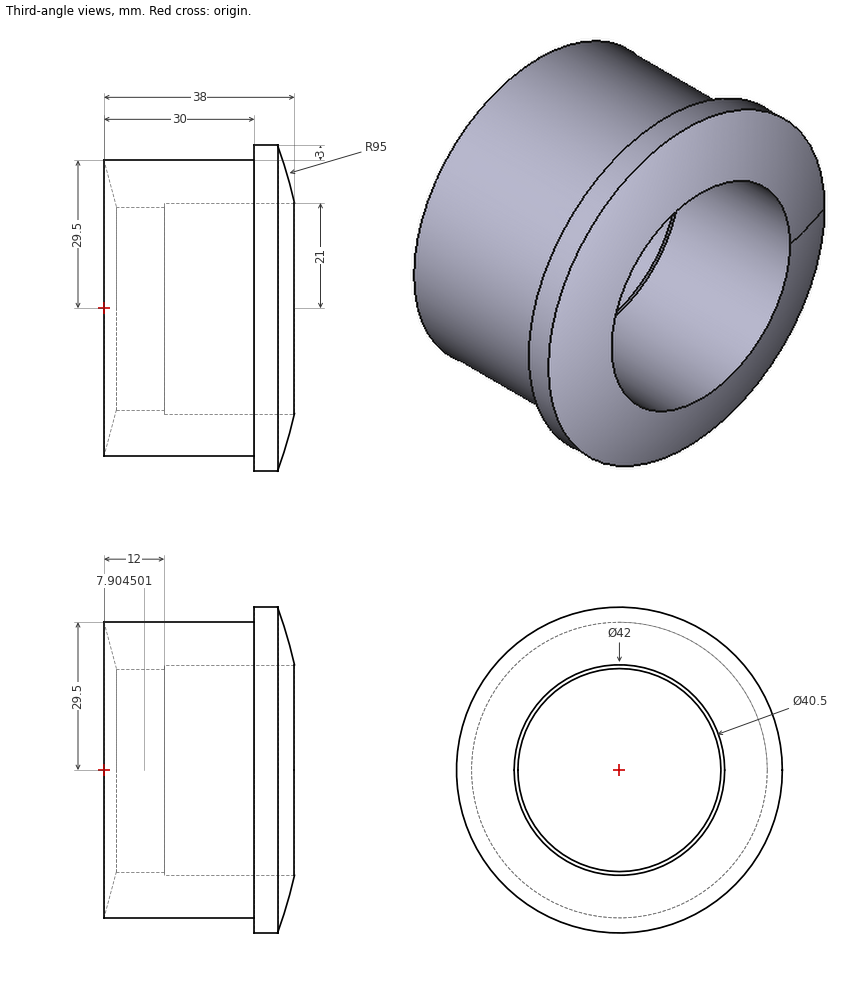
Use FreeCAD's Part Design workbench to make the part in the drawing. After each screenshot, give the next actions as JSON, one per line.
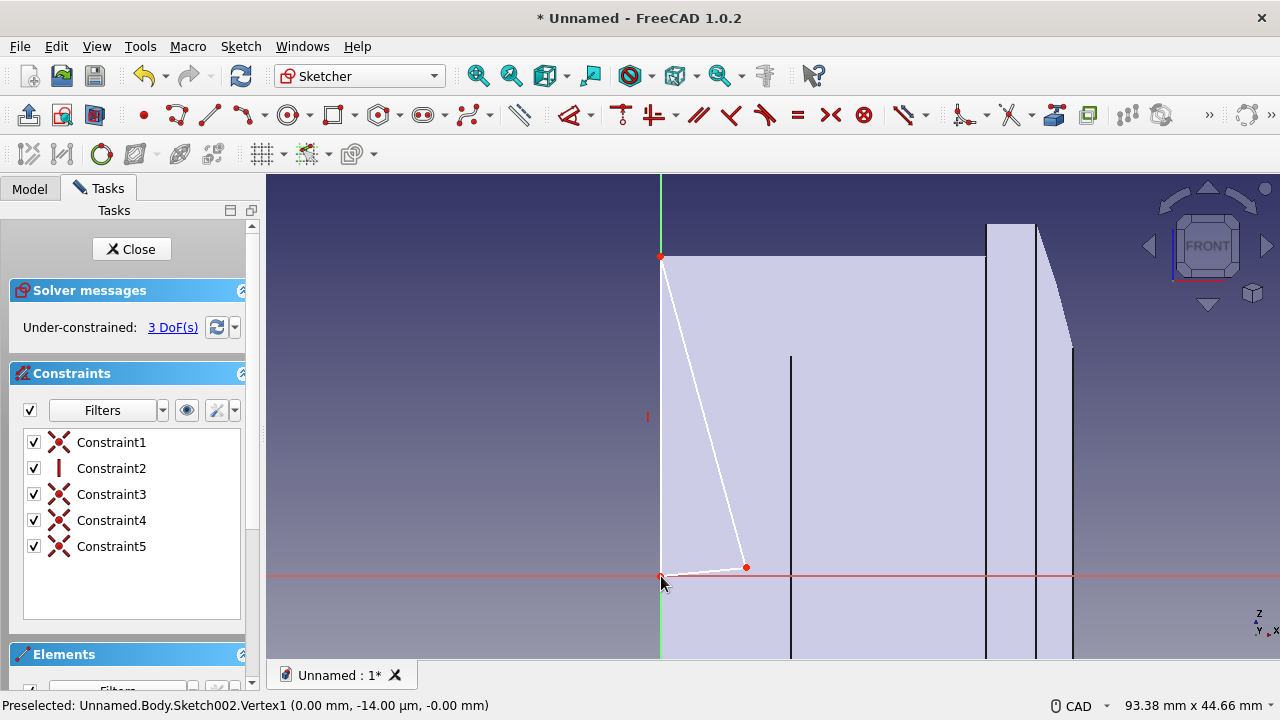
{"action": "left_click", "coordinate": [686, 574]}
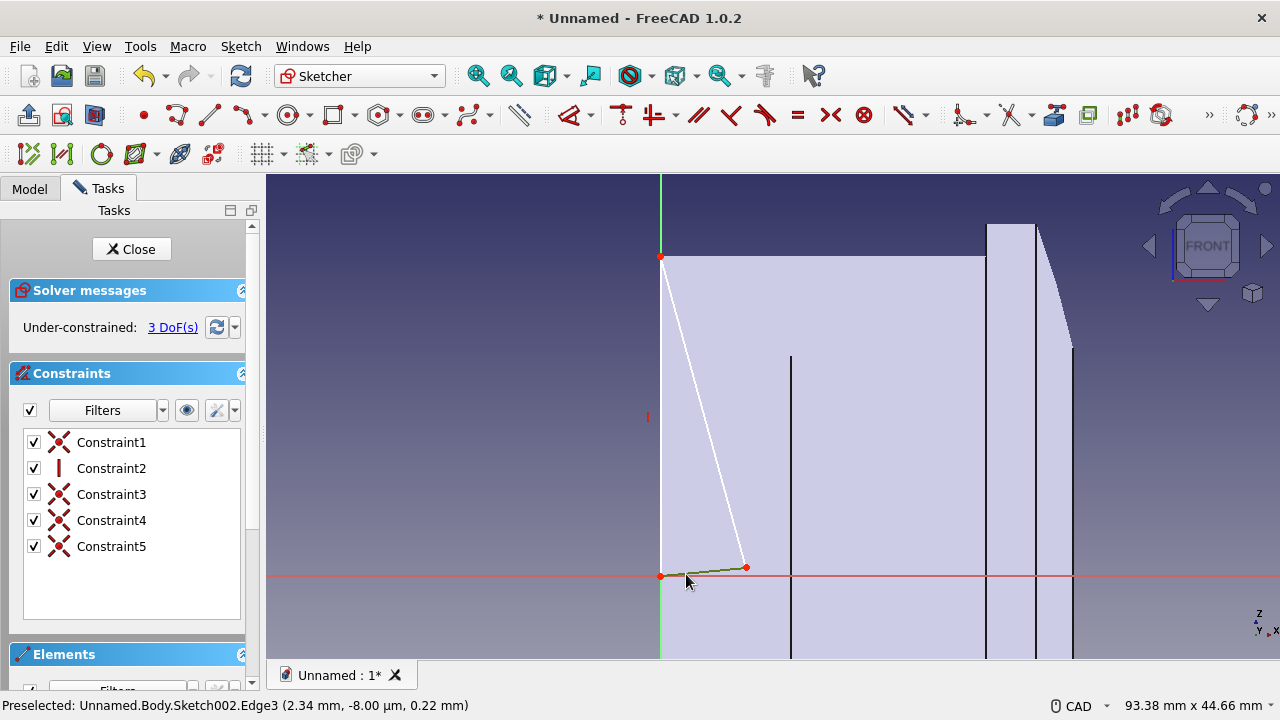
{"action": "left_click", "coordinate": [676, 116]}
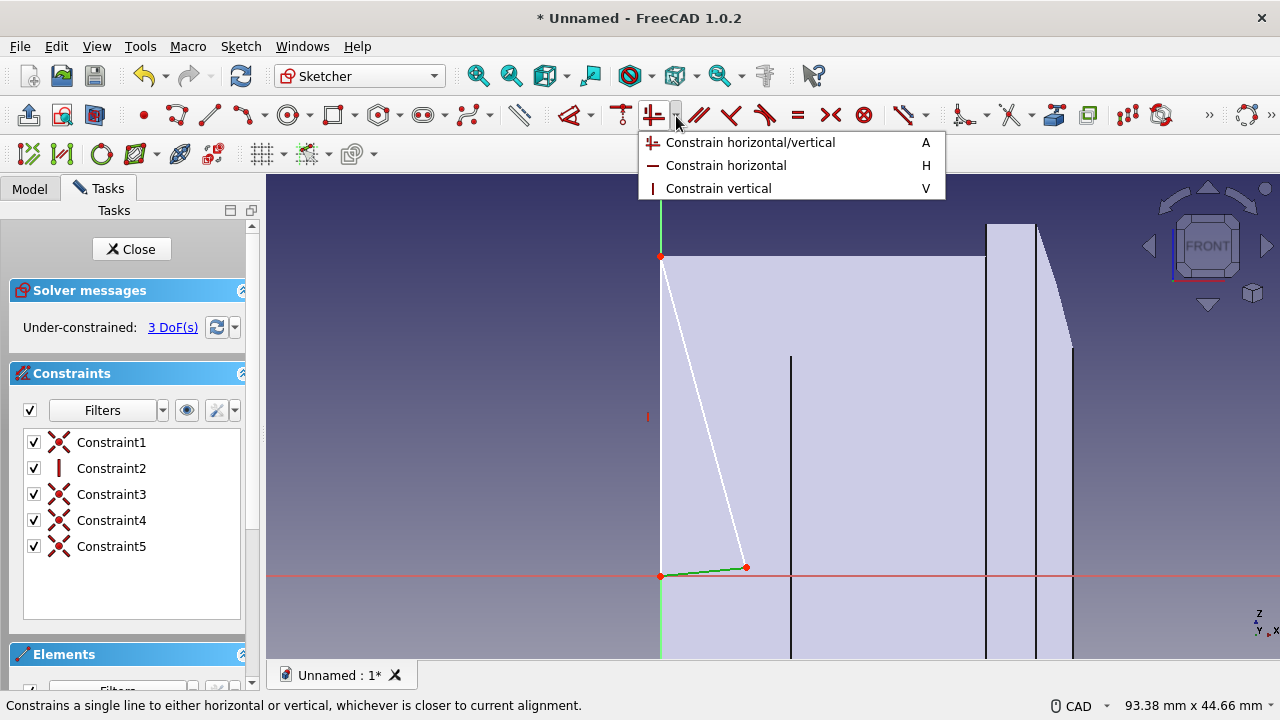
{"action": "left_click", "coordinate": [792, 166]}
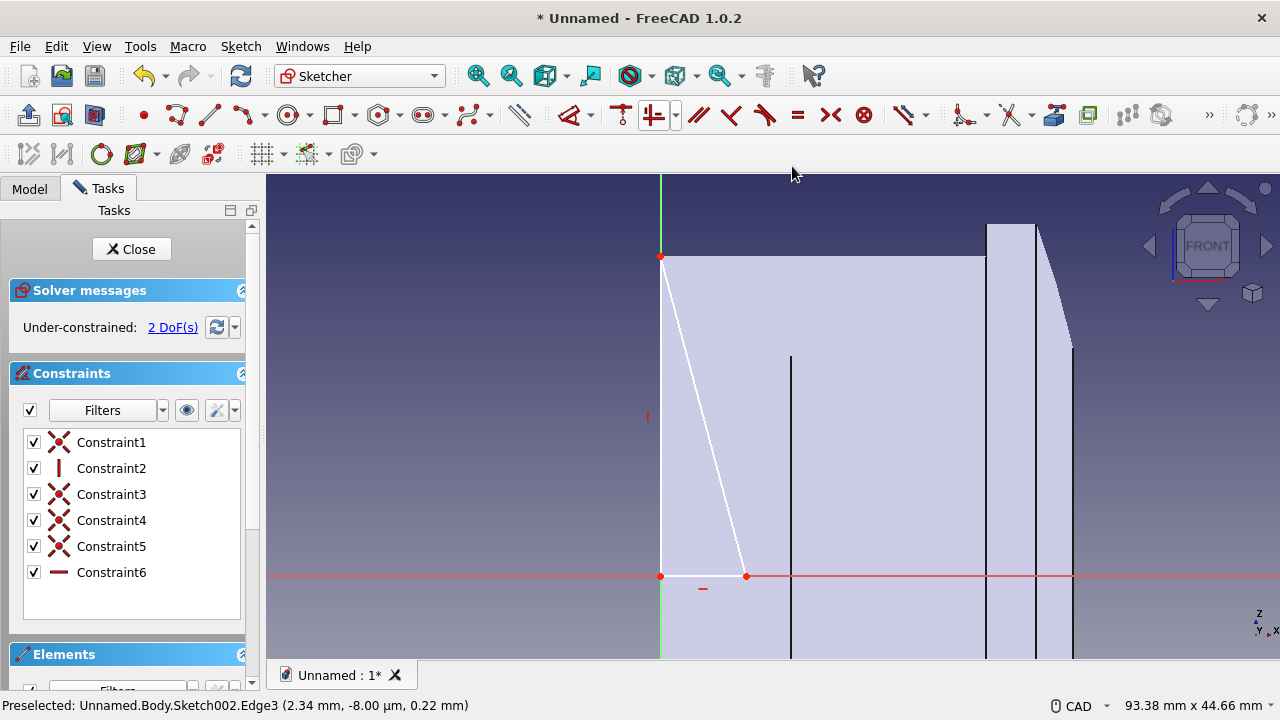
{"action": "left_click", "coordinate": [568, 116]}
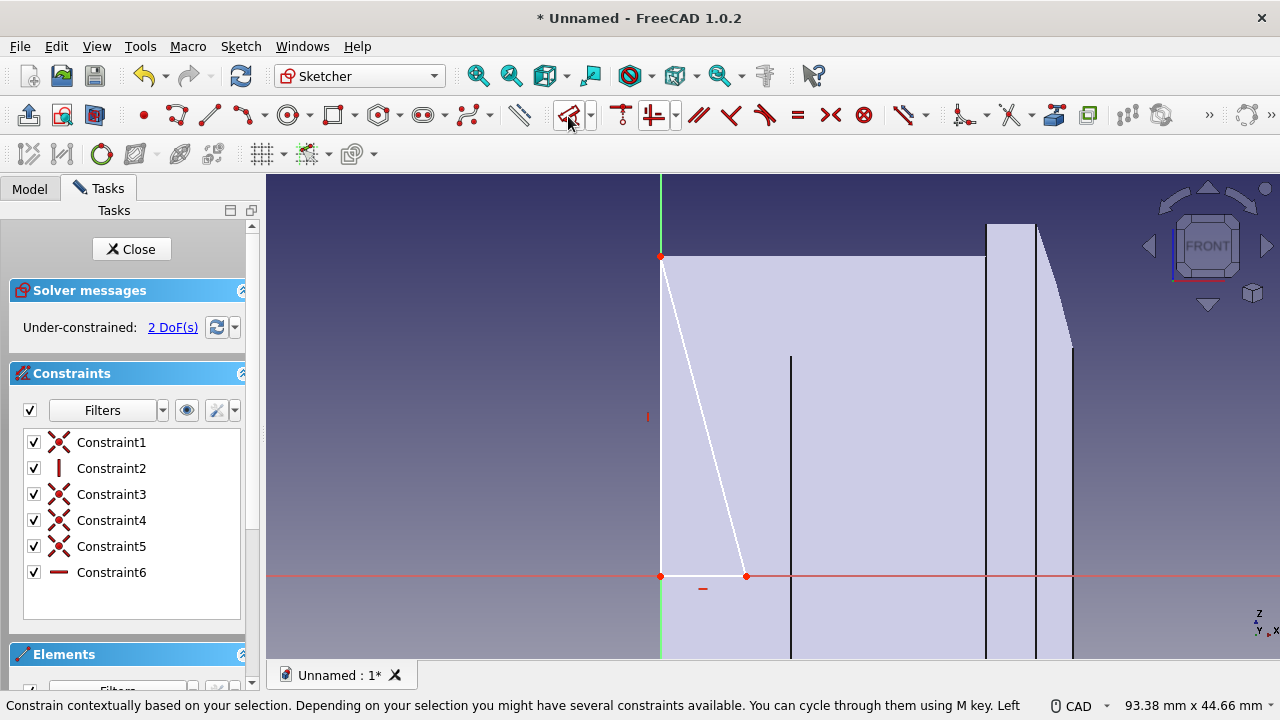
{"action": "left_click", "coordinate": [661, 480]}
{"action": "left_click", "coordinate": [627, 417]}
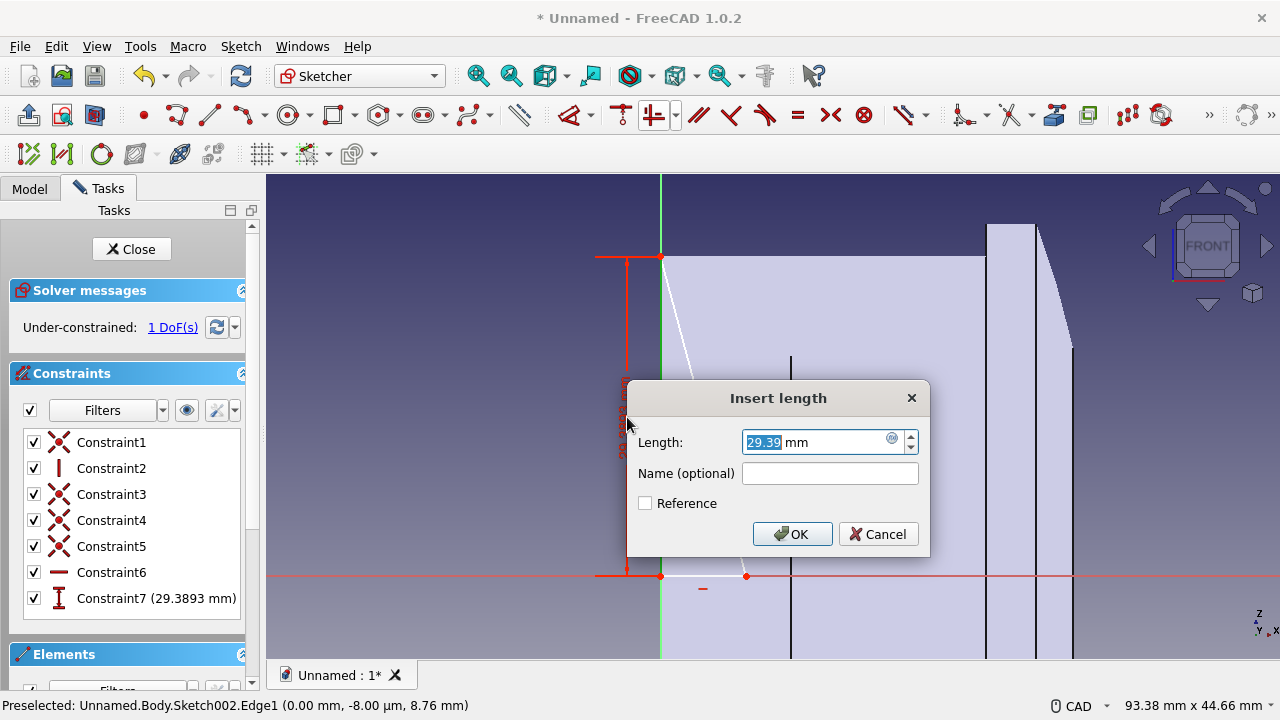
{"action": "type", "text": "29.5"}
{"action": "key", "text": "Return"}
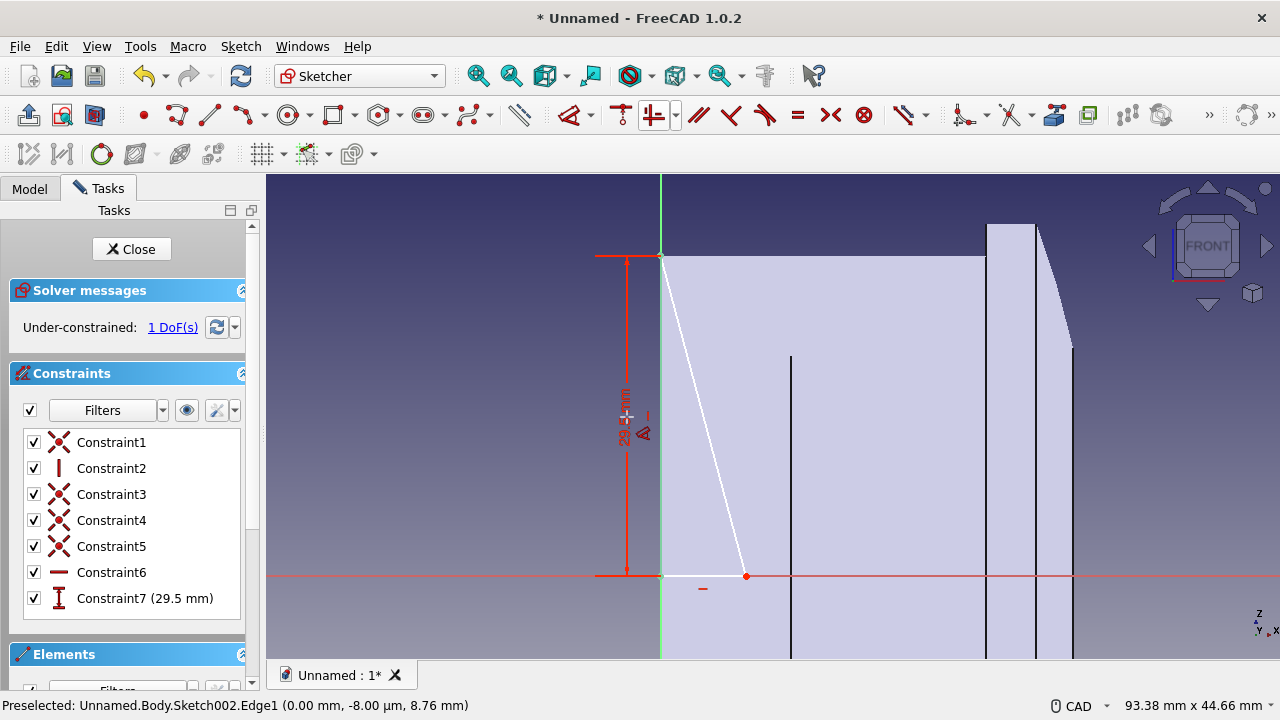
{"action": "left_click", "coordinate": [720, 576]}
{"action": "left_click", "coordinate": [703, 610]}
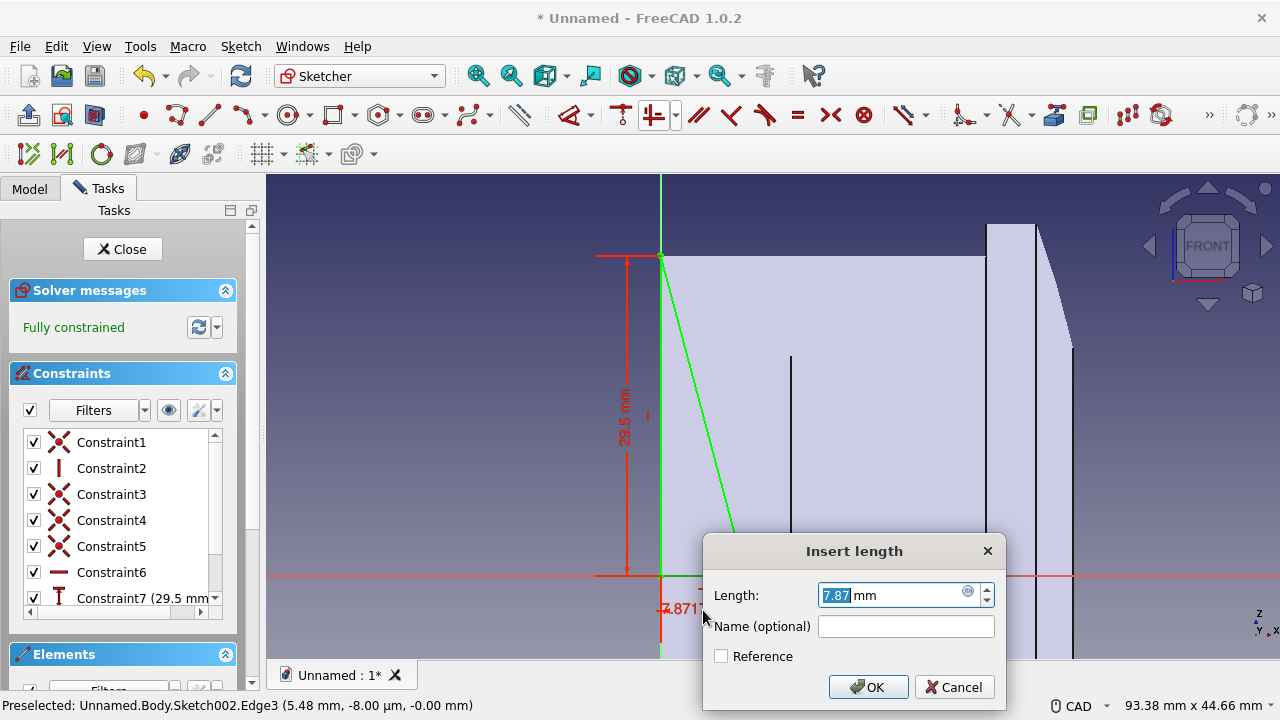
{"action": "type", "text": "7.904501"}
{"action": "key", "text": "Return"}
{"action": "key", "text": "Escape"}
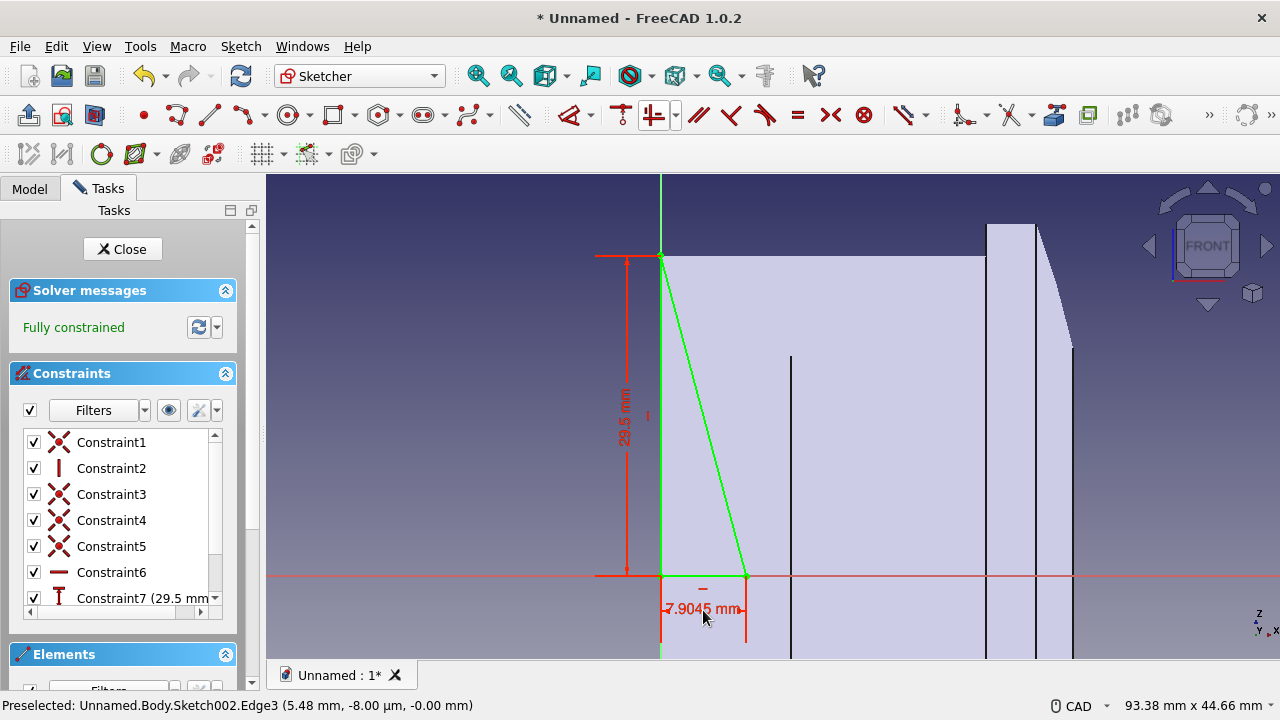
{"action": "left_click", "coordinate": [123, 249]}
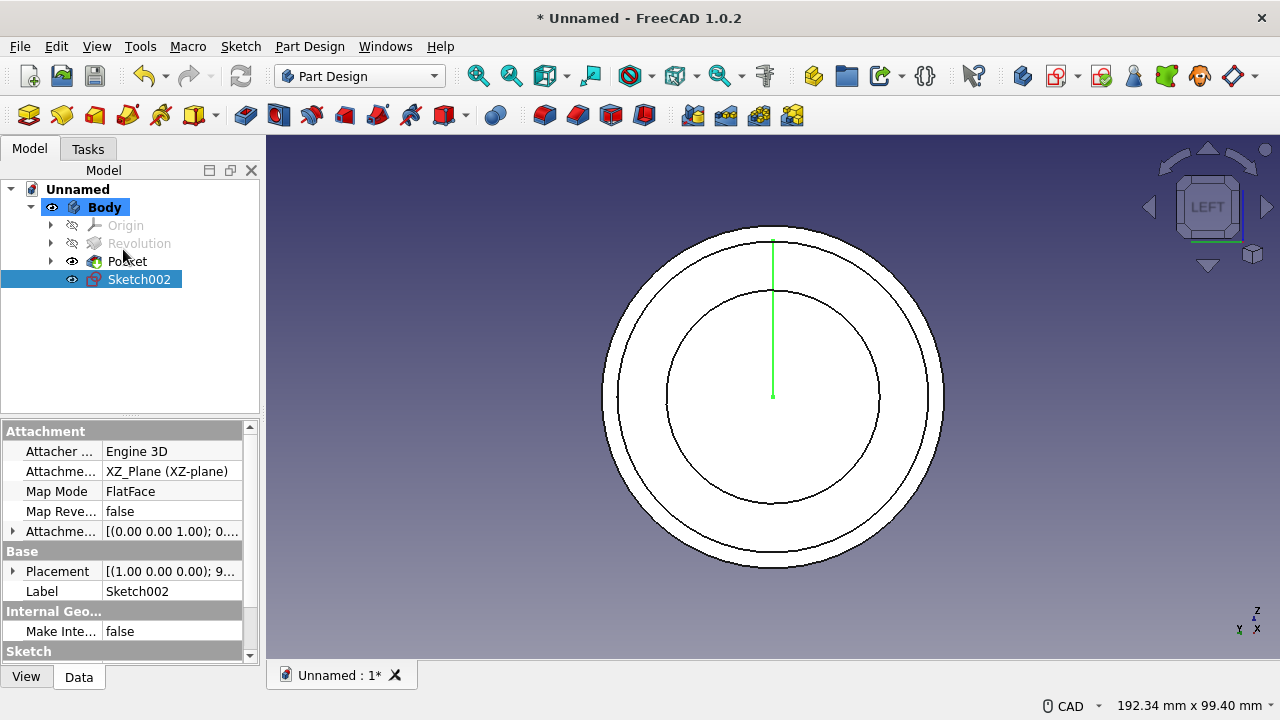
{"action": "left_click", "coordinate": [312, 116]}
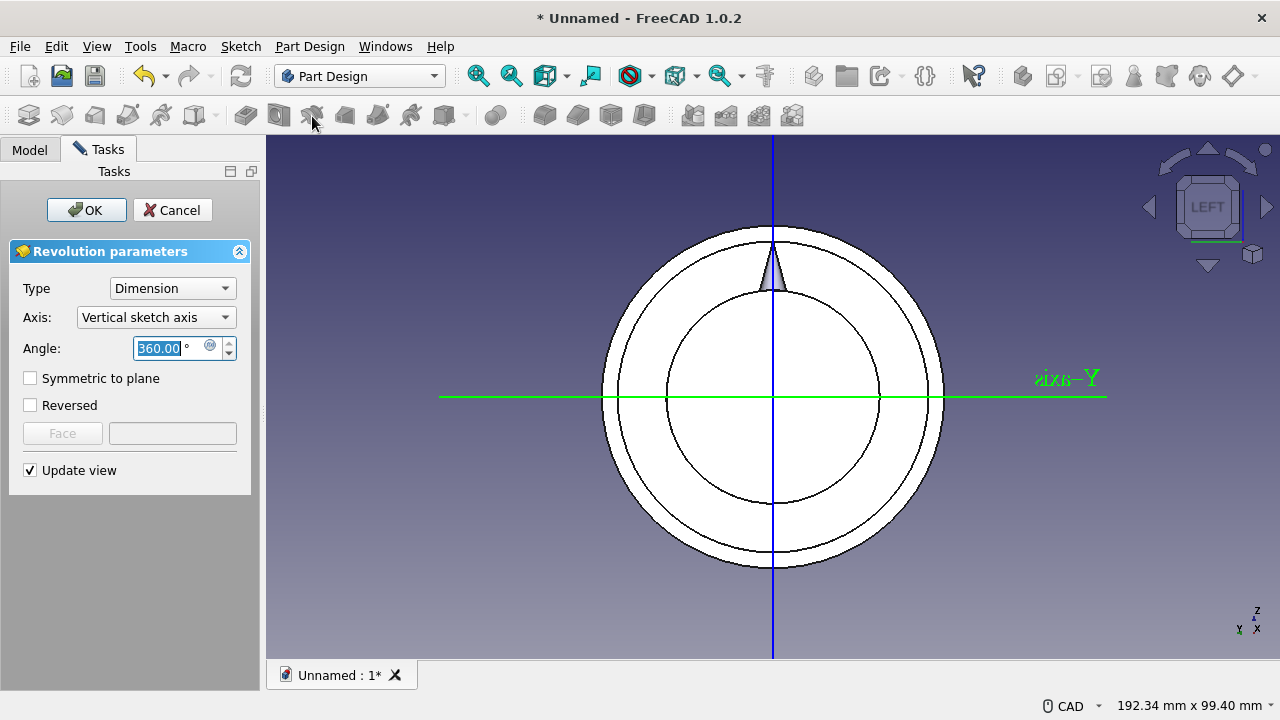
{"action": "left_click", "coordinate": [157, 318]}